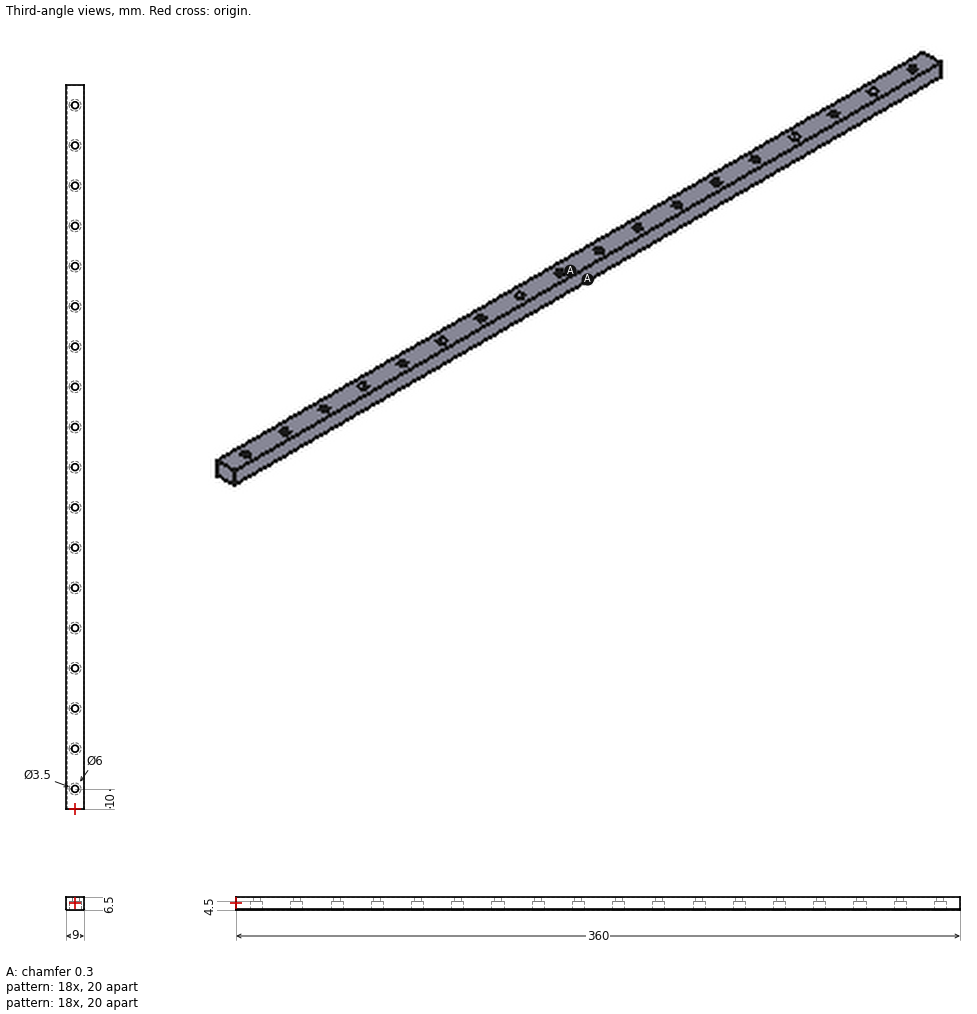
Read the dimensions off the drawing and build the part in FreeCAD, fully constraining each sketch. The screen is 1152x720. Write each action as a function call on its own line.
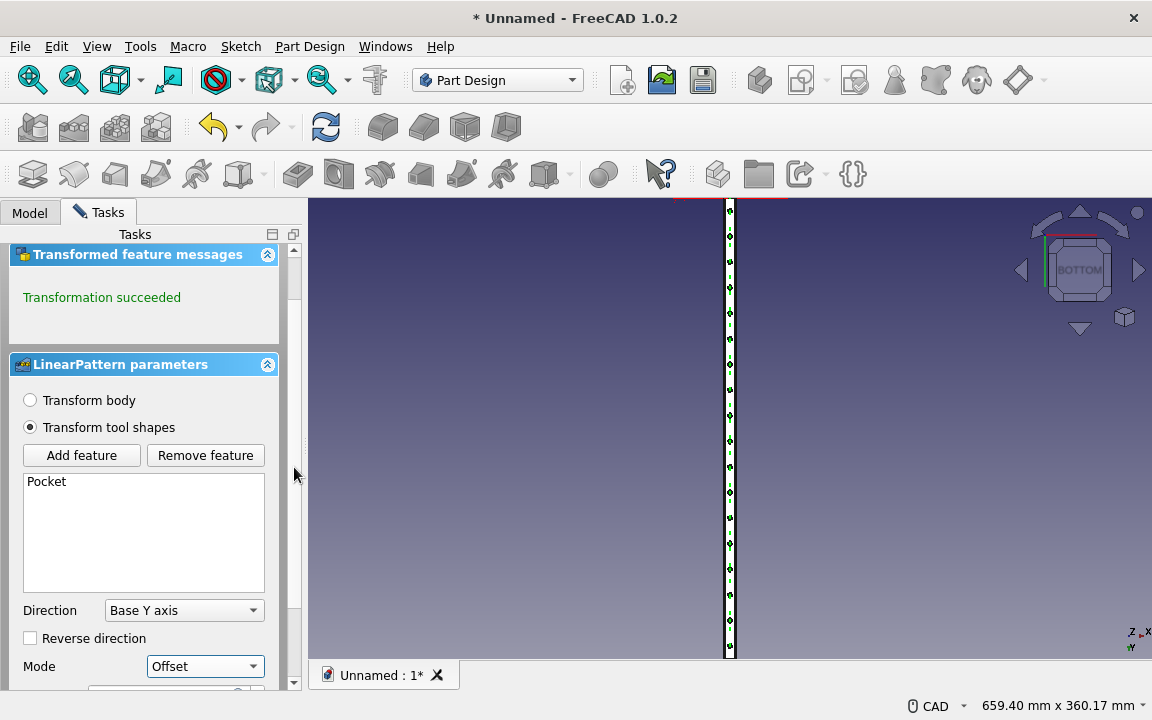
click(101, 273)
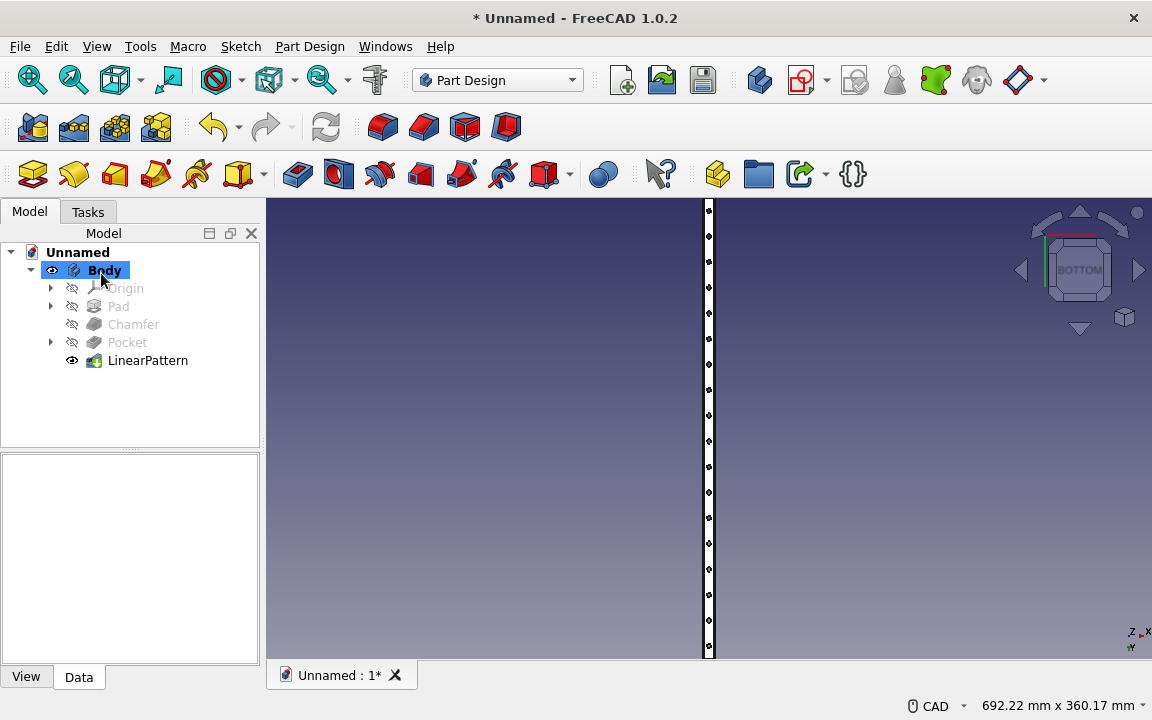
key(v)
key(f)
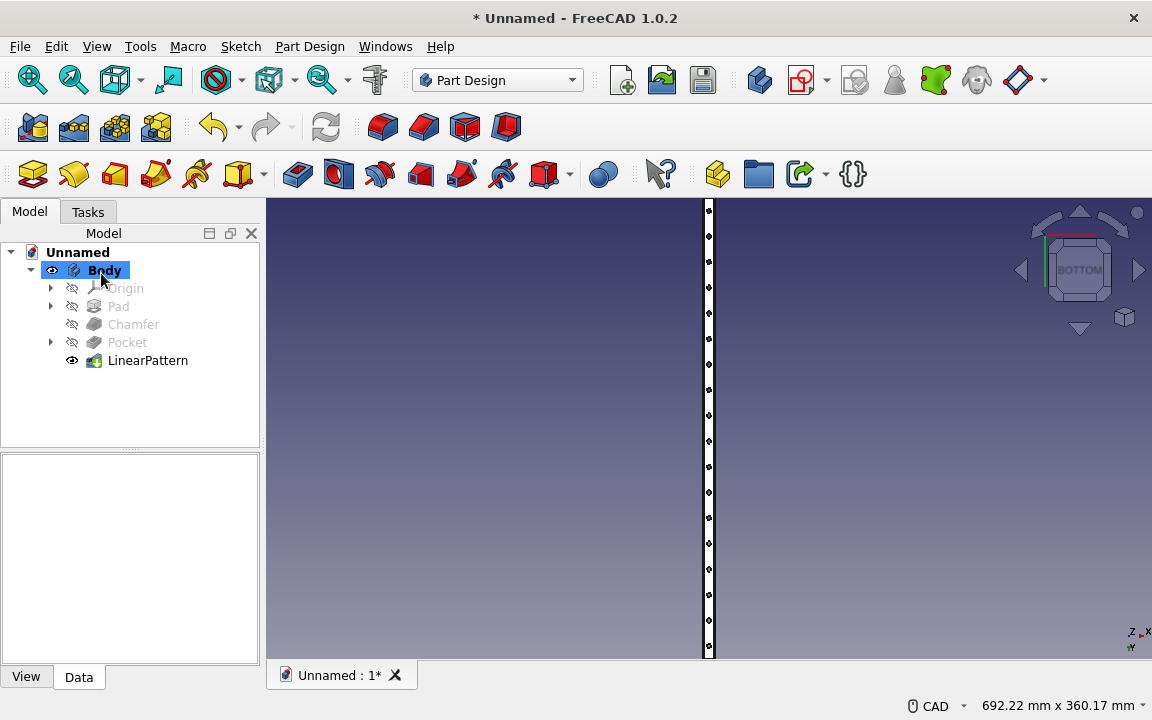
scroll(709, 559, up, 5)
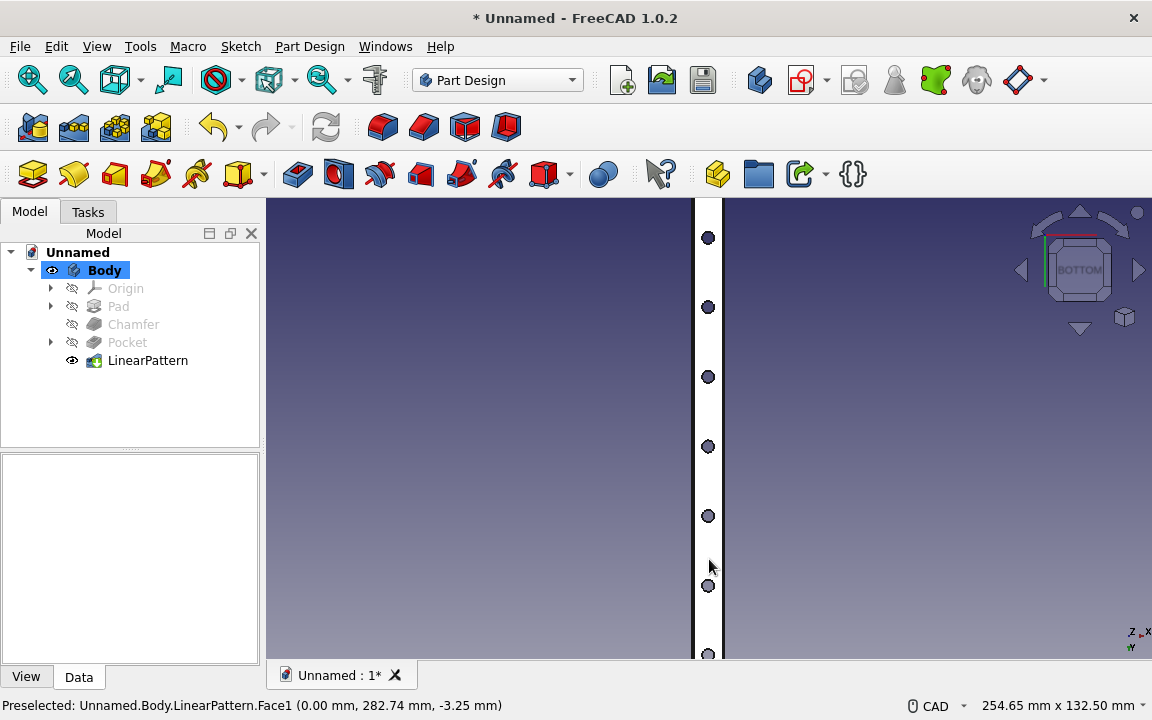
click(708, 560)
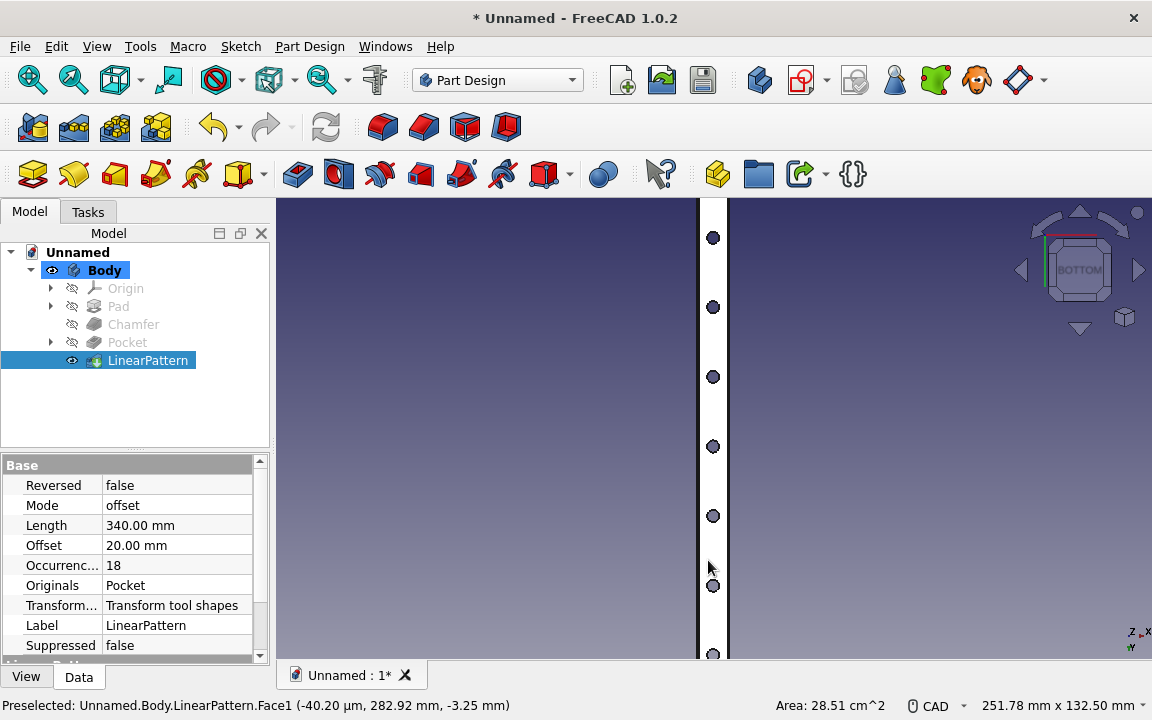
click(800, 80)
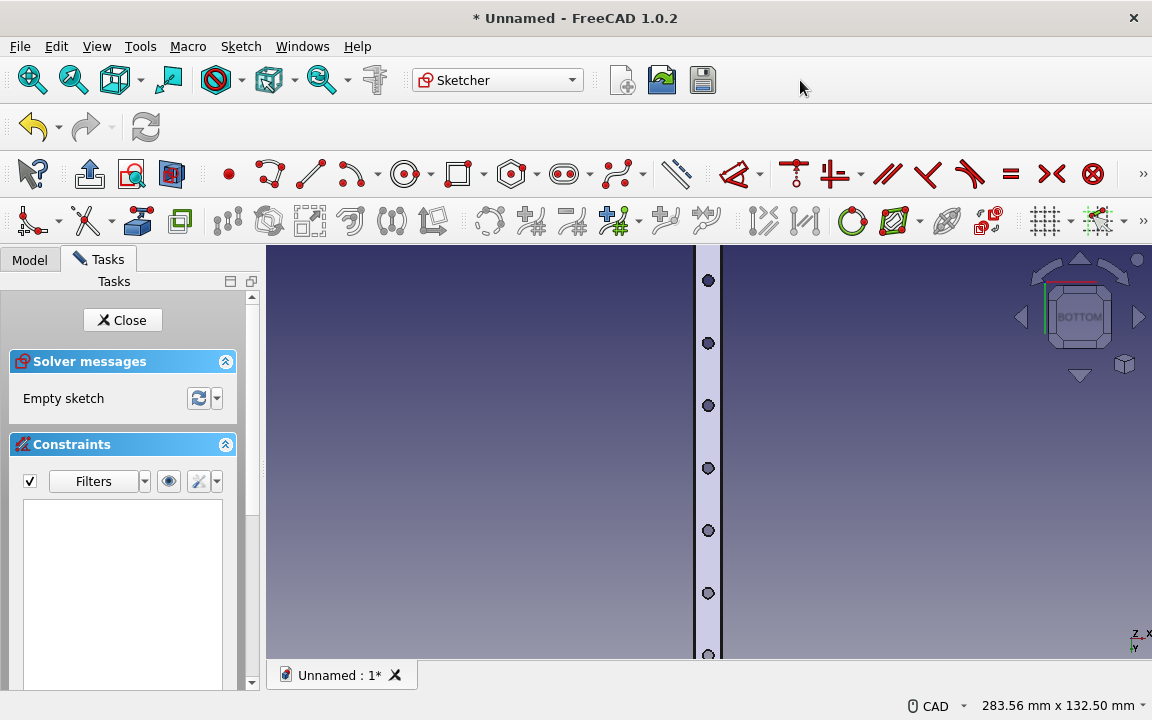
scroll(640, 452, down, 5)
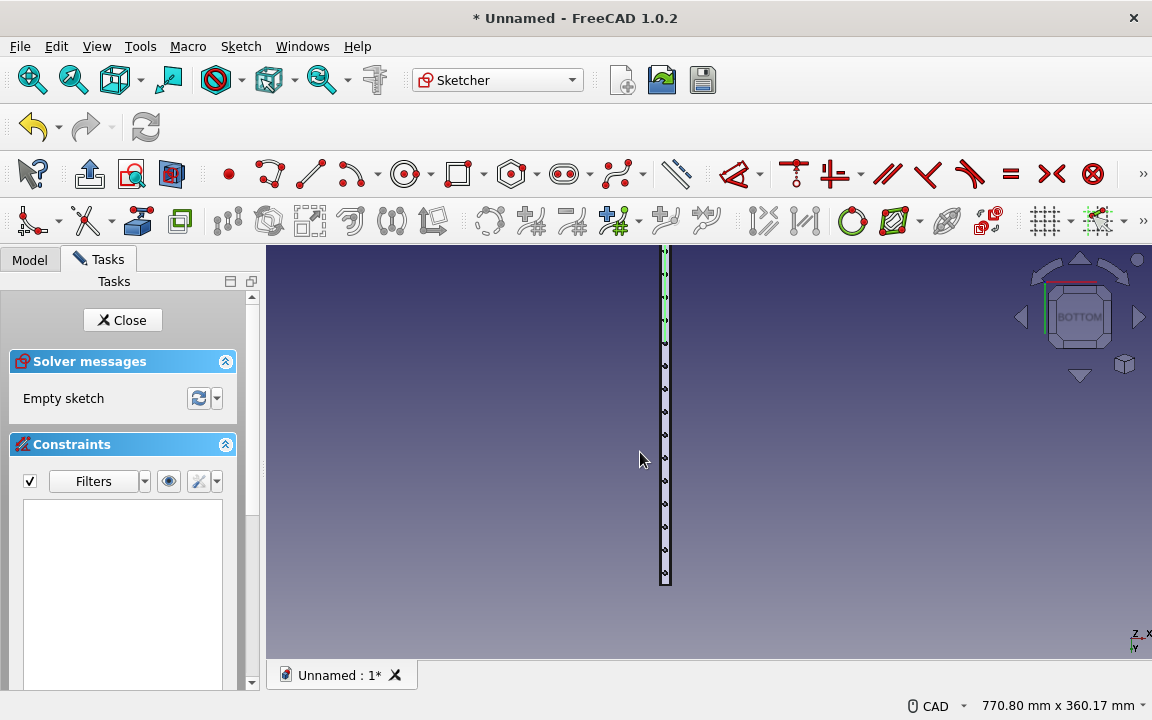
scroll(640, 452, down, 5)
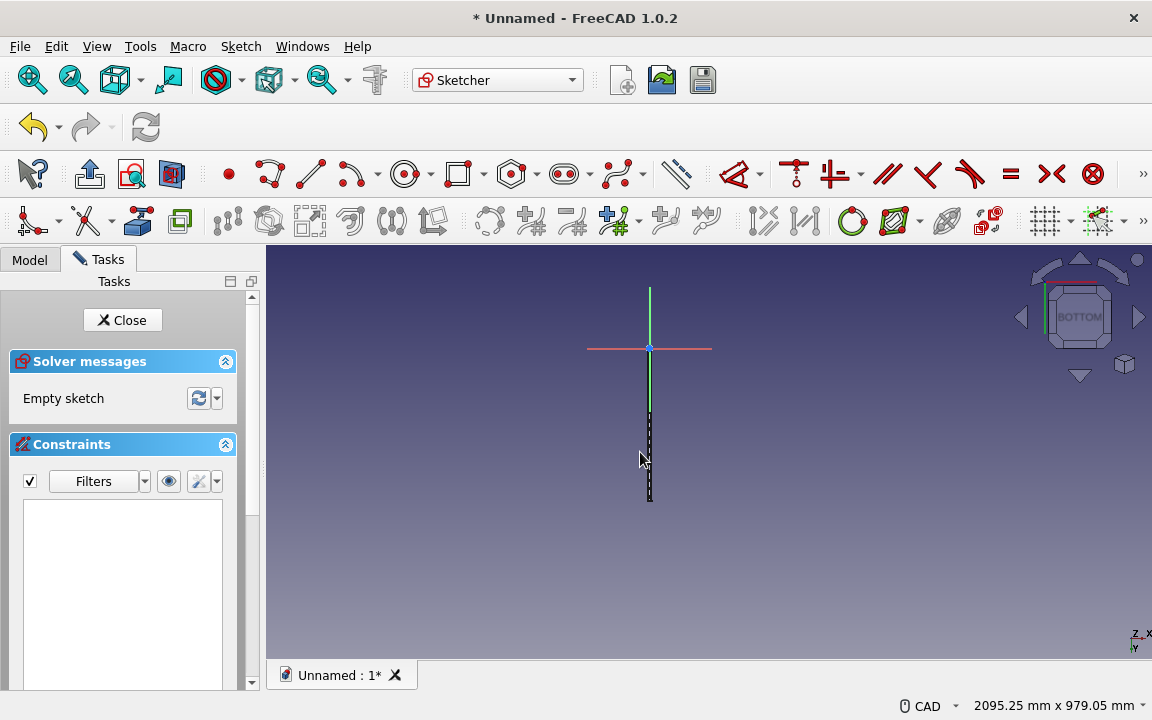
scroll(650, 346, up, 15)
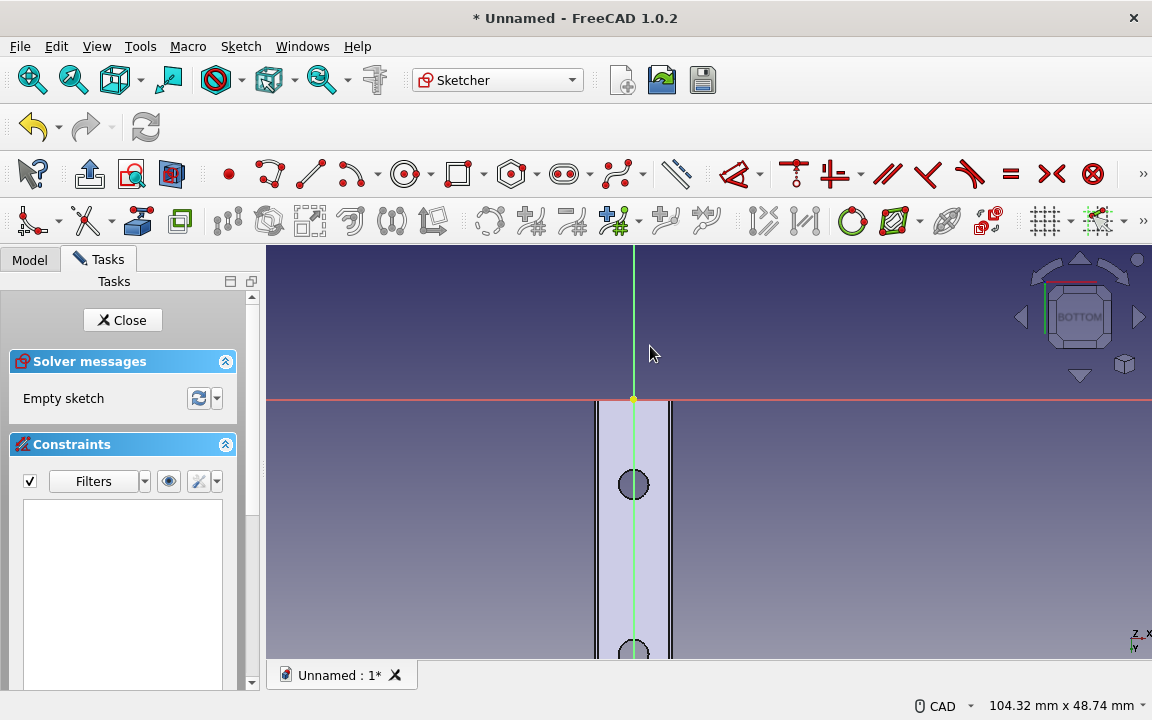
scroll(628, 457, up, 4)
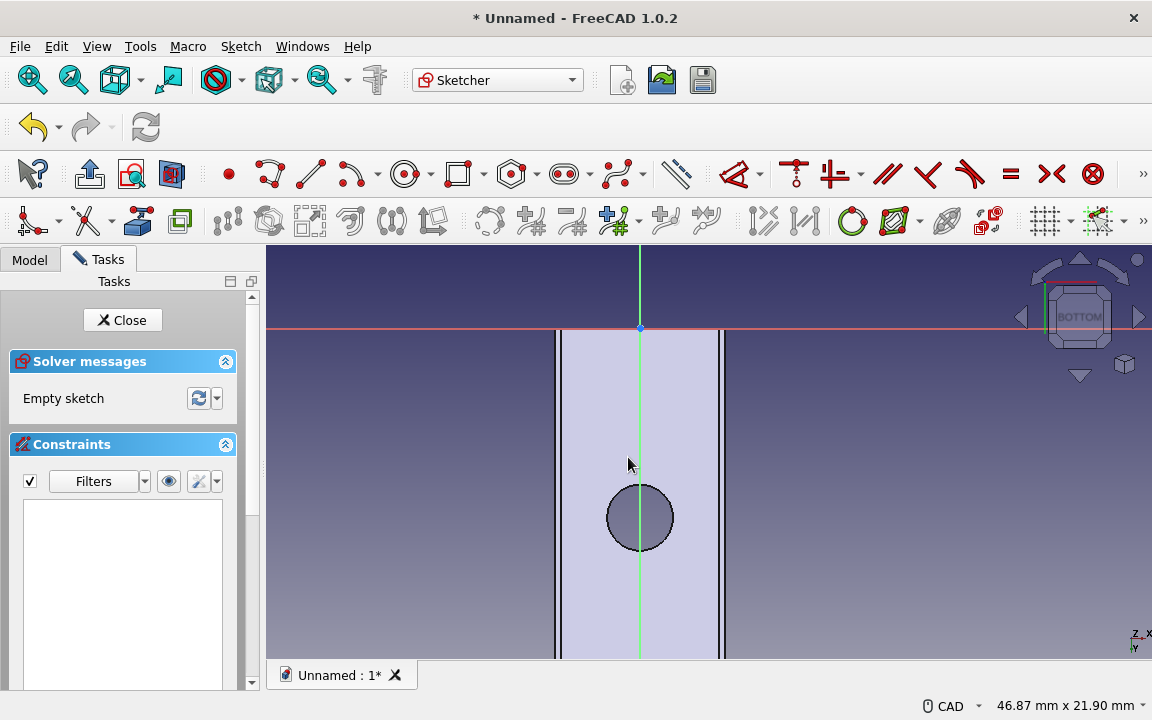
key(g)
key(c)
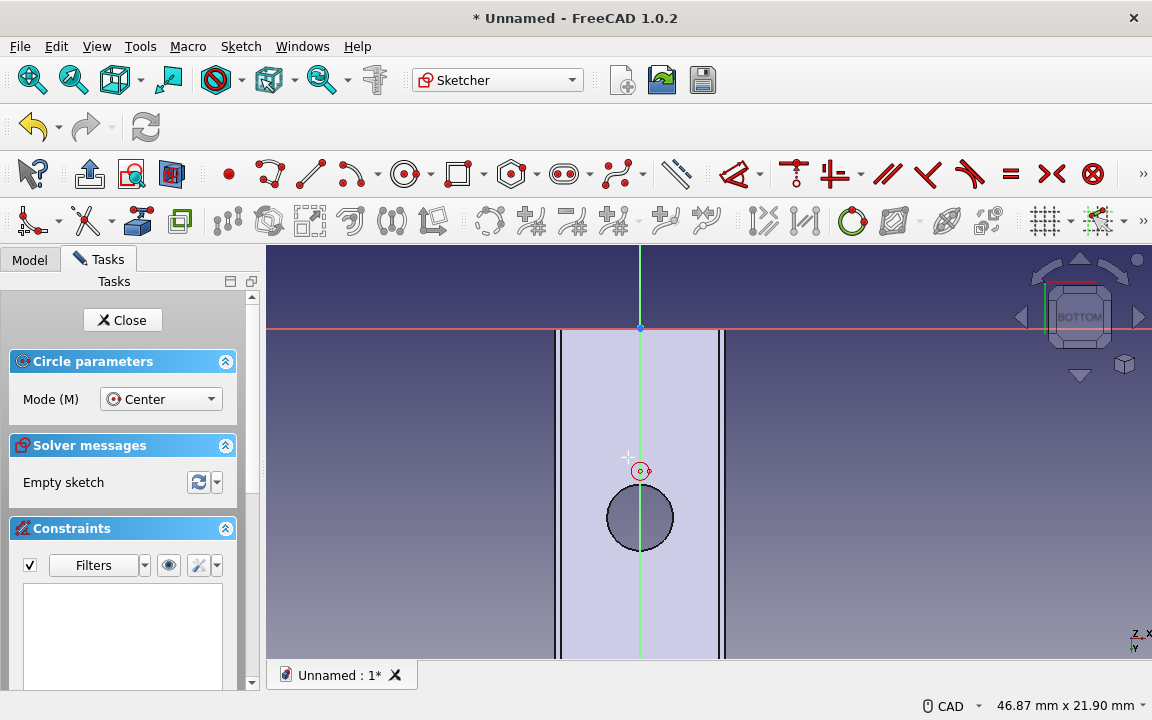
click(640, 518)
move(680, 478)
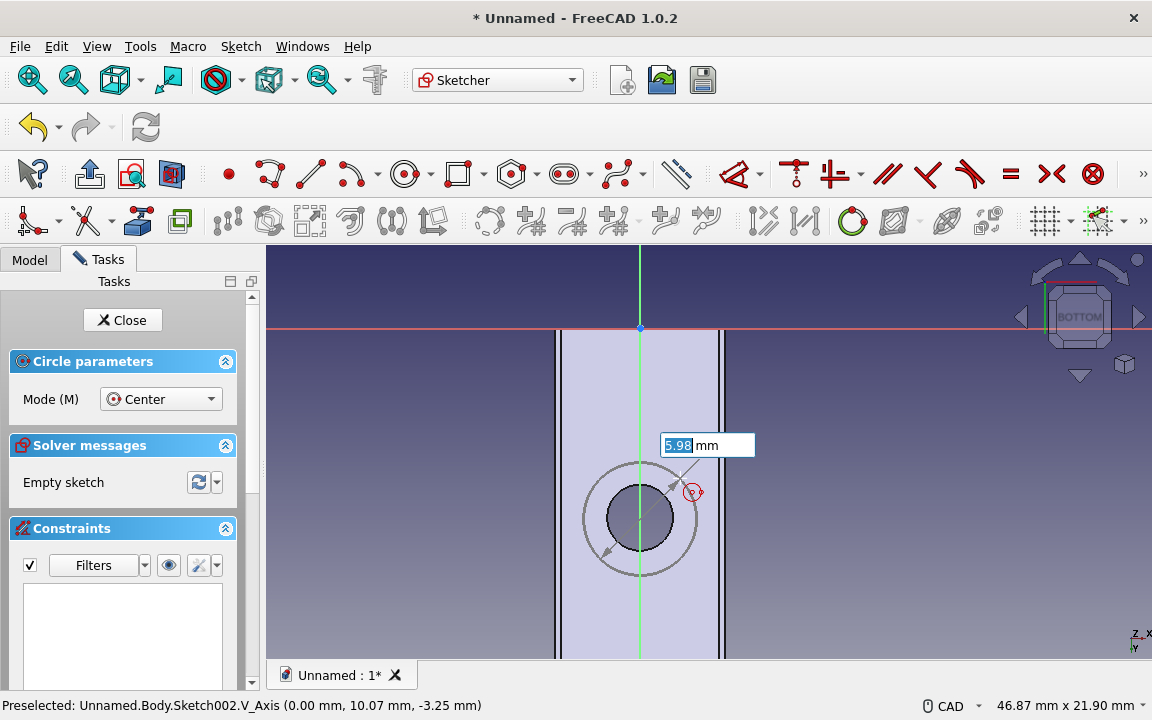
text(6)
key(Return)
key(Escape)